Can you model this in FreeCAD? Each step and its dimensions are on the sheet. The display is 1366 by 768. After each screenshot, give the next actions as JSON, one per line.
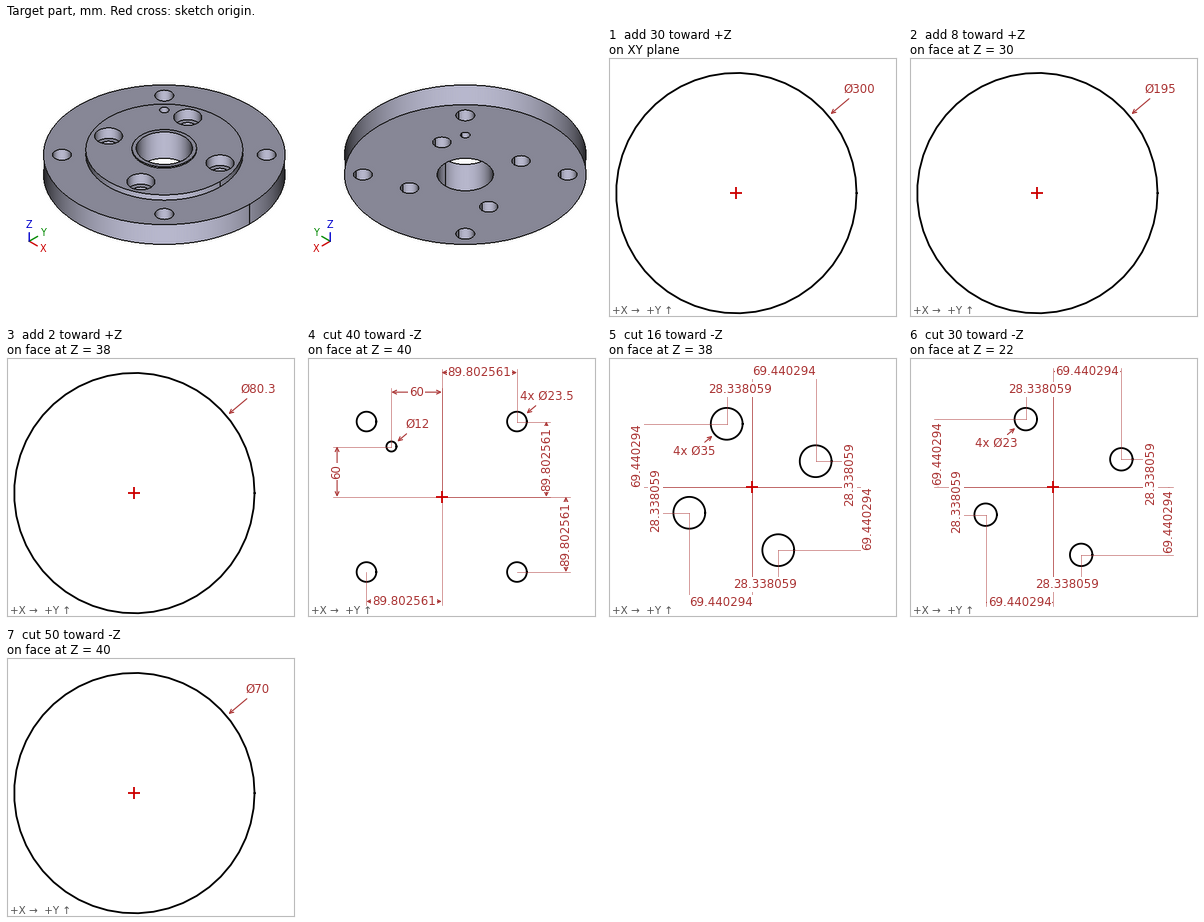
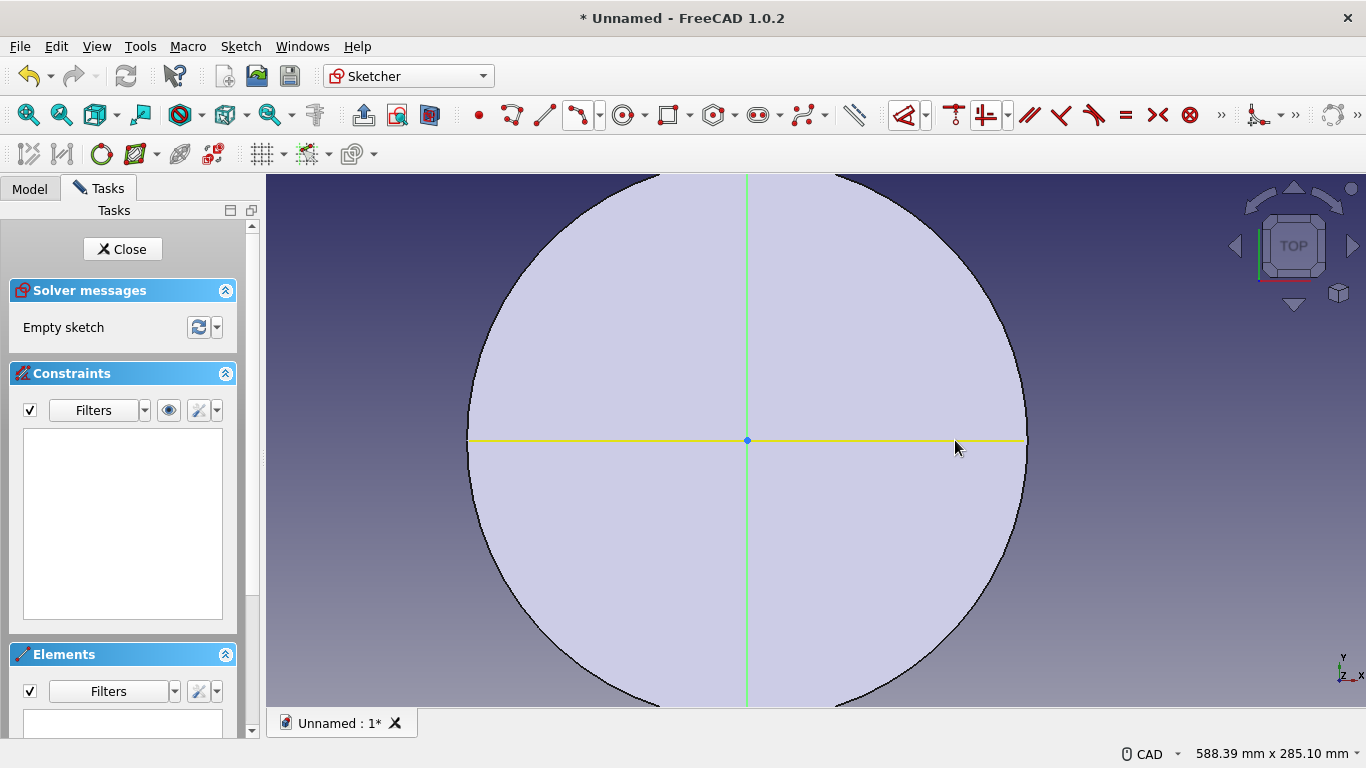
{"action": "key", "text": "g c"}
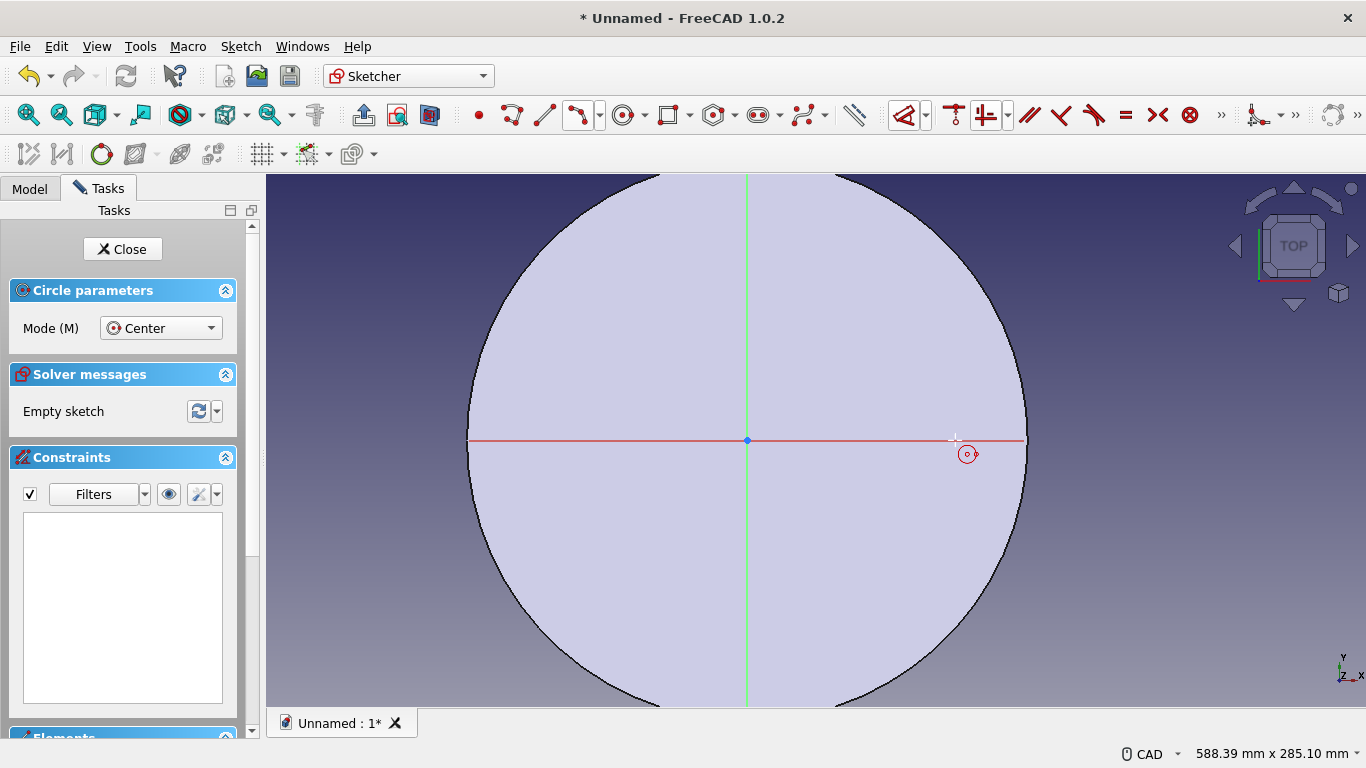
{"action": "left_click", "coordinate": [747, 440]}
{"action": "left_click", "coordinate": [876, 312]}
{"action": "key", "text": "Escape"}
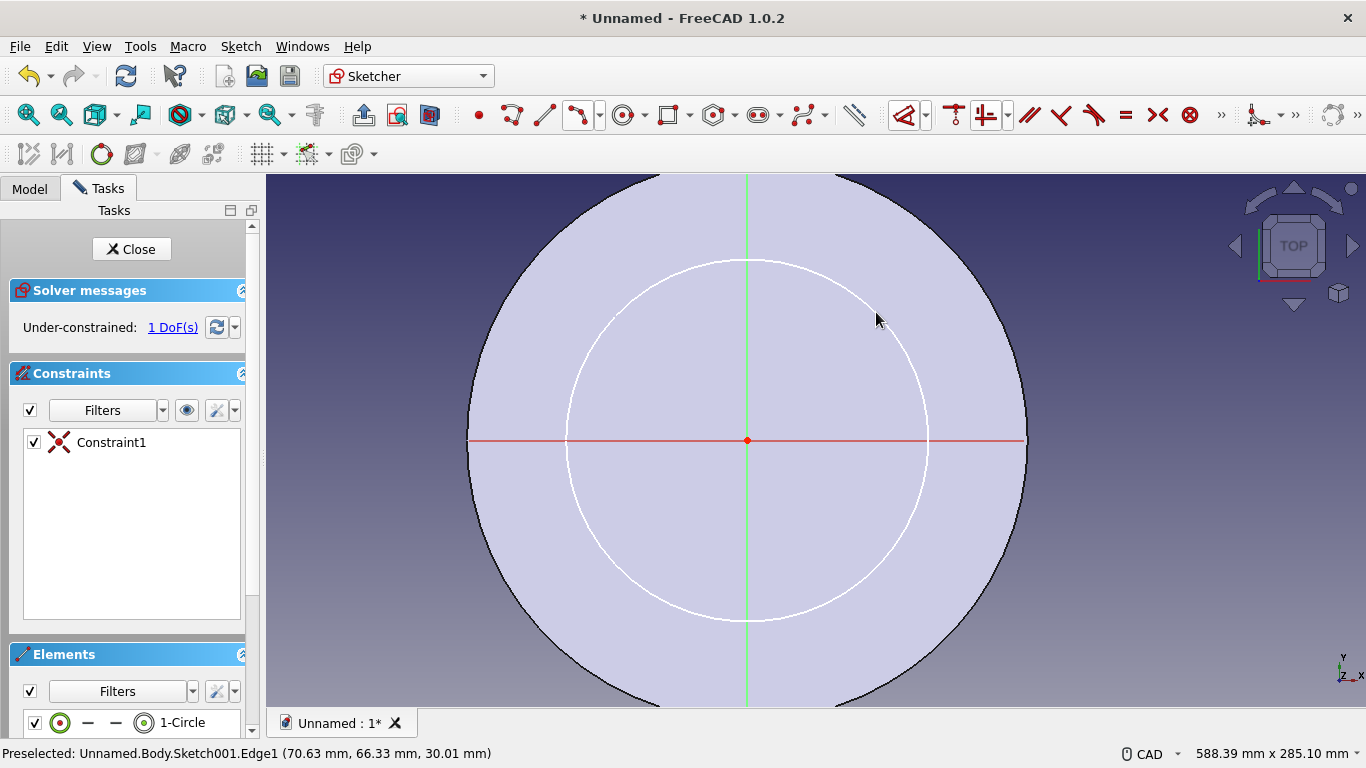
{"action": "left_click", "coordinate": [904, 116]}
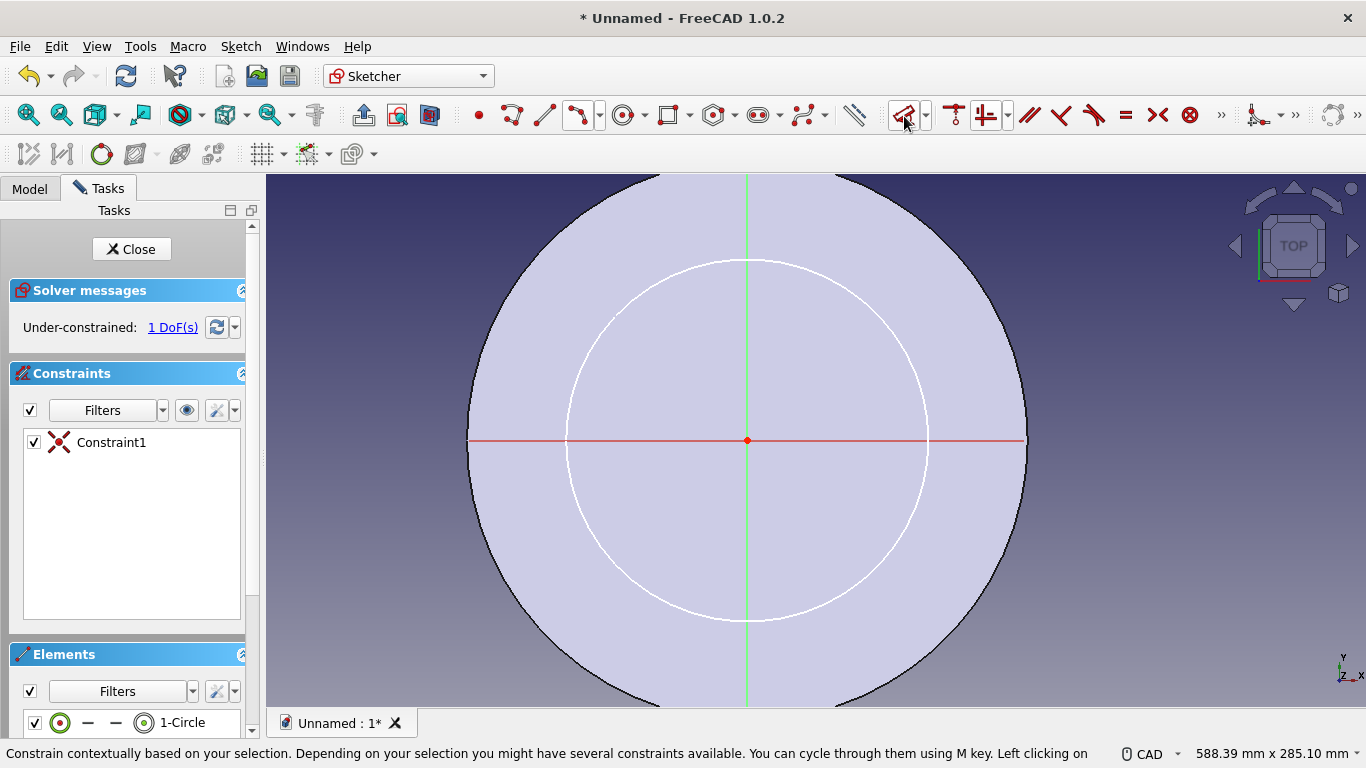
{"action": "left_click", "coordinate": [875, 312]}
{"action": "left_click", "coordinate": [898, 289]}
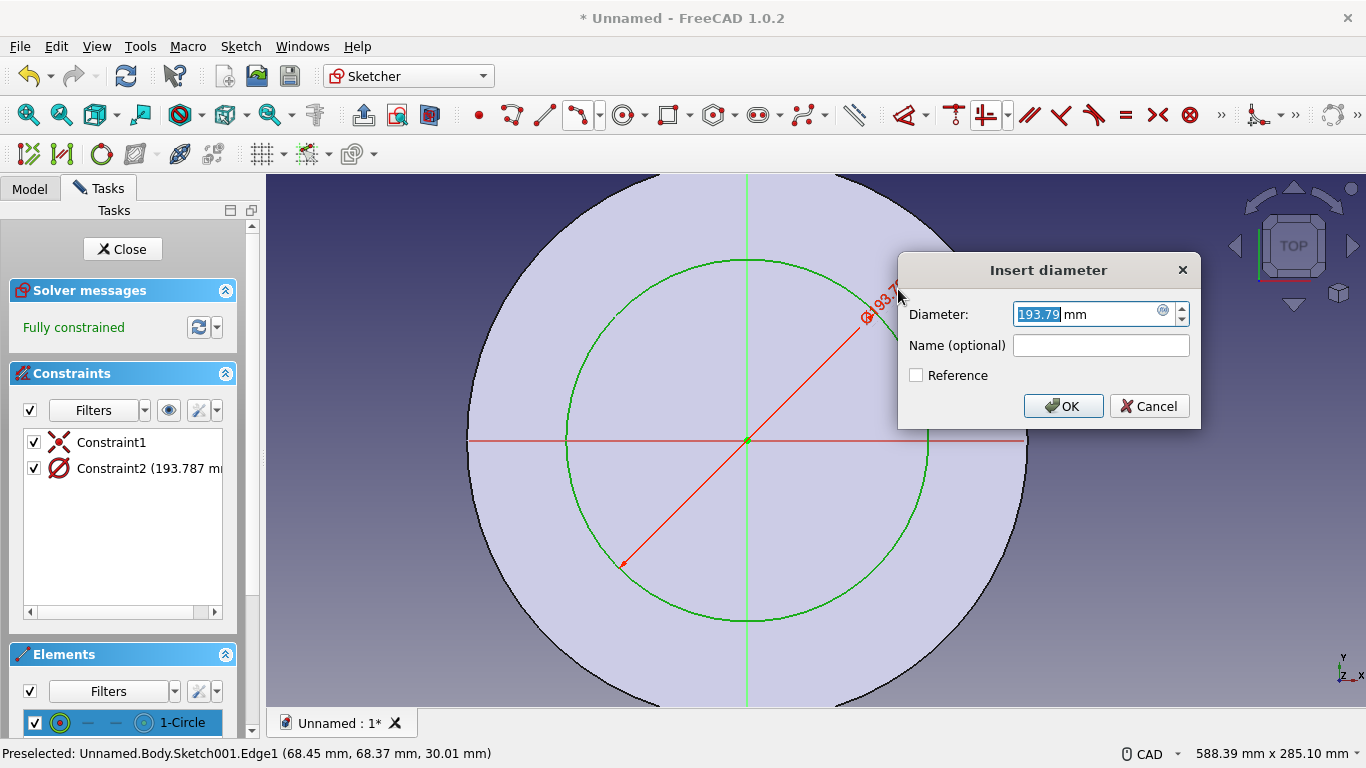
{"action": "type", "text": "195"}
{"action": "key", "text": "Return"}
{"action": "key", "text": "Escape"}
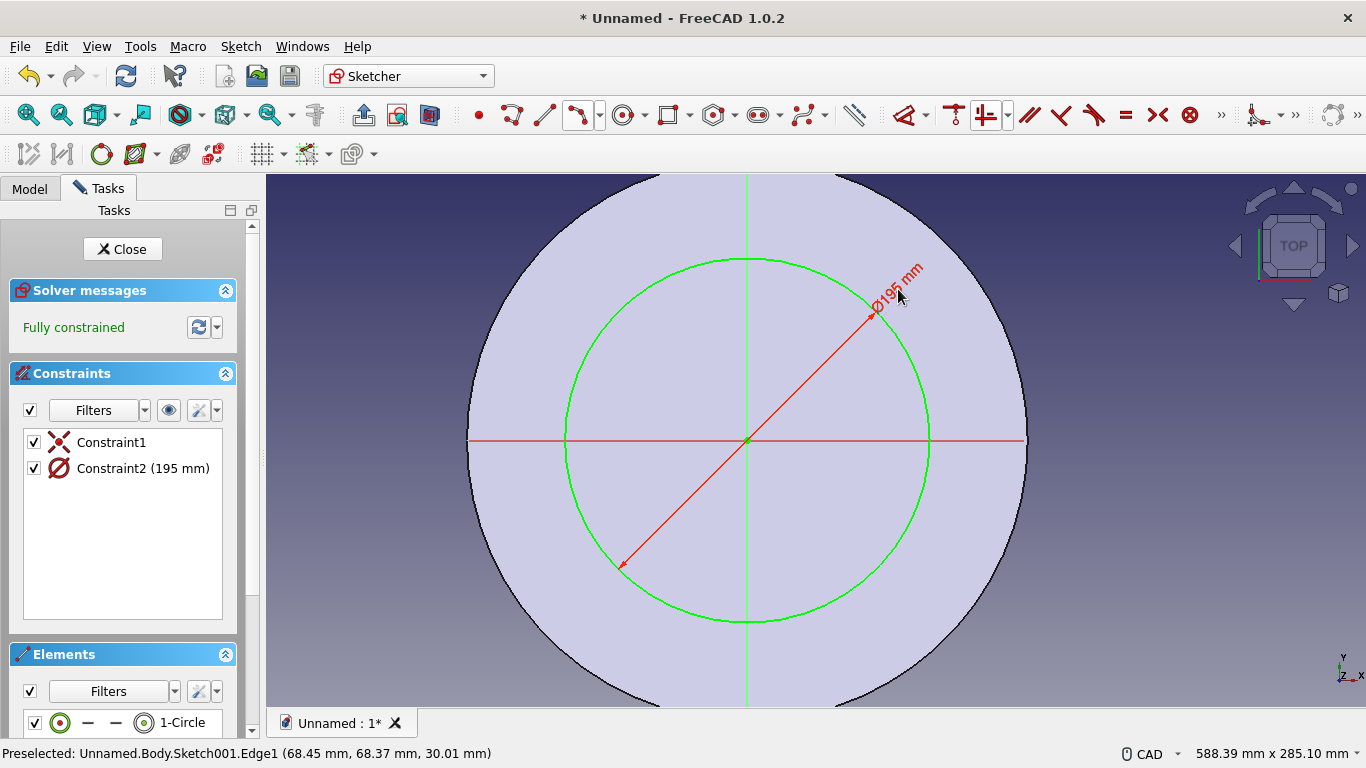
{"action": "left_click", "coordinate": [123, 249]}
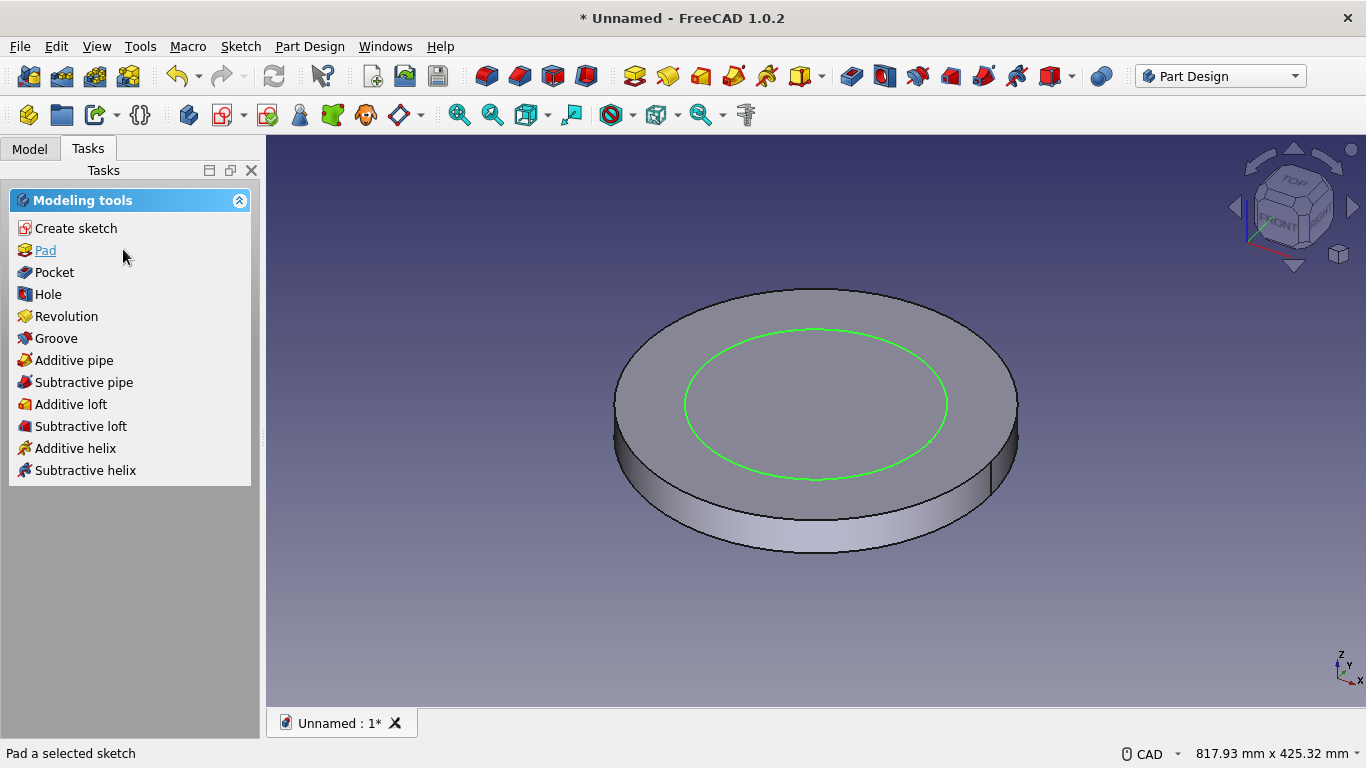
{"action": "left_click", "coordinate": [635, 76]}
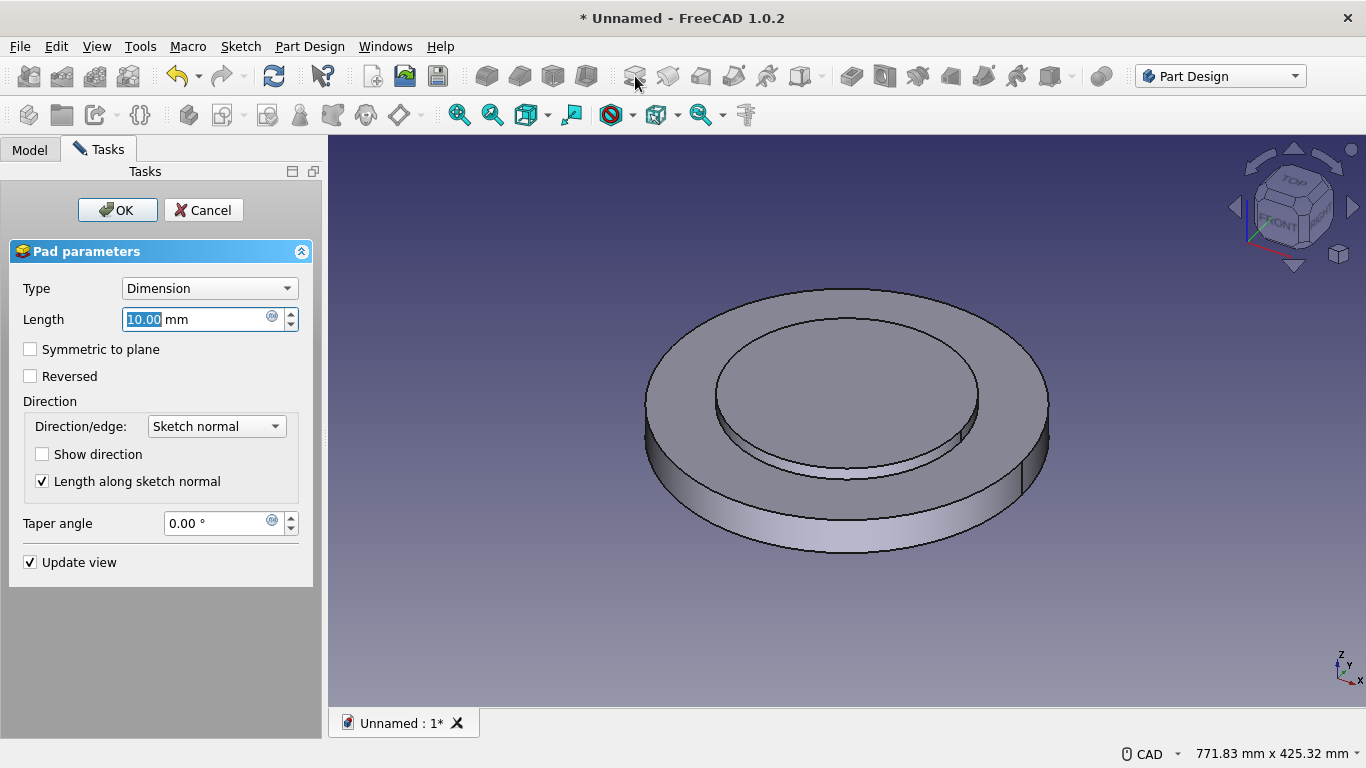
{"action": "type", "text": "8"}
{"action": "key", "text": "Tab"}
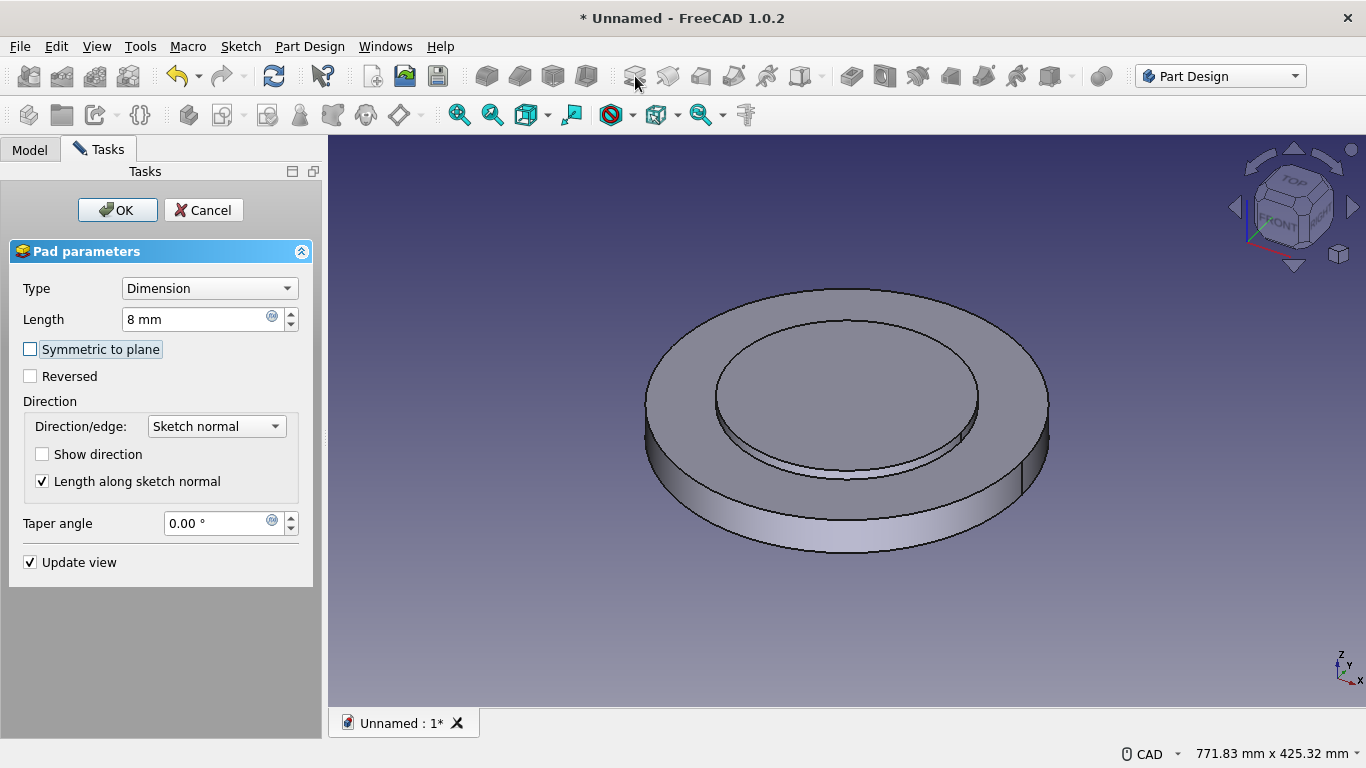
{"action": "left_click", "coordinate": [118, 210]}